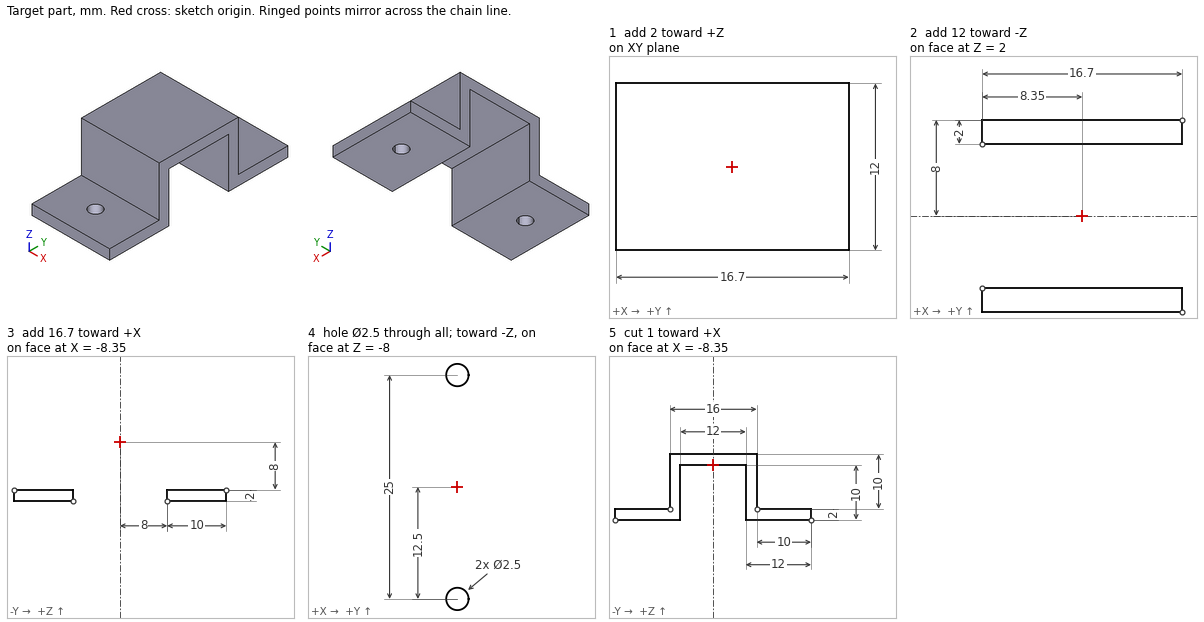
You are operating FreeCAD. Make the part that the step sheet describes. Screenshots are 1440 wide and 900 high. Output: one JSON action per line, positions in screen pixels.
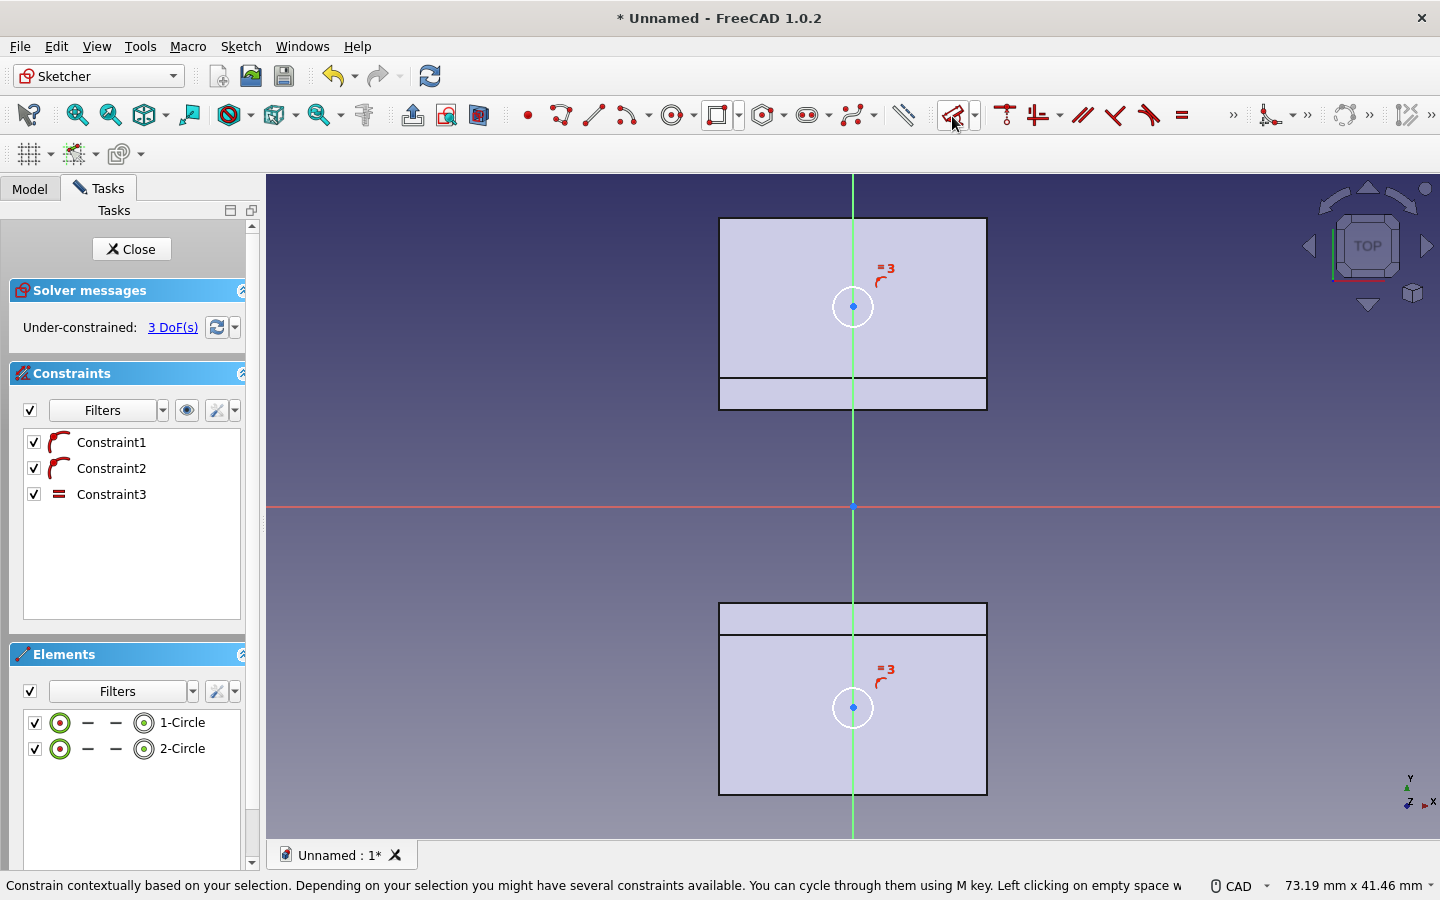
{"action": "left_click", "coordinate": [867, 694]}
{"action": "left_click", "coordinate": [890, 671]}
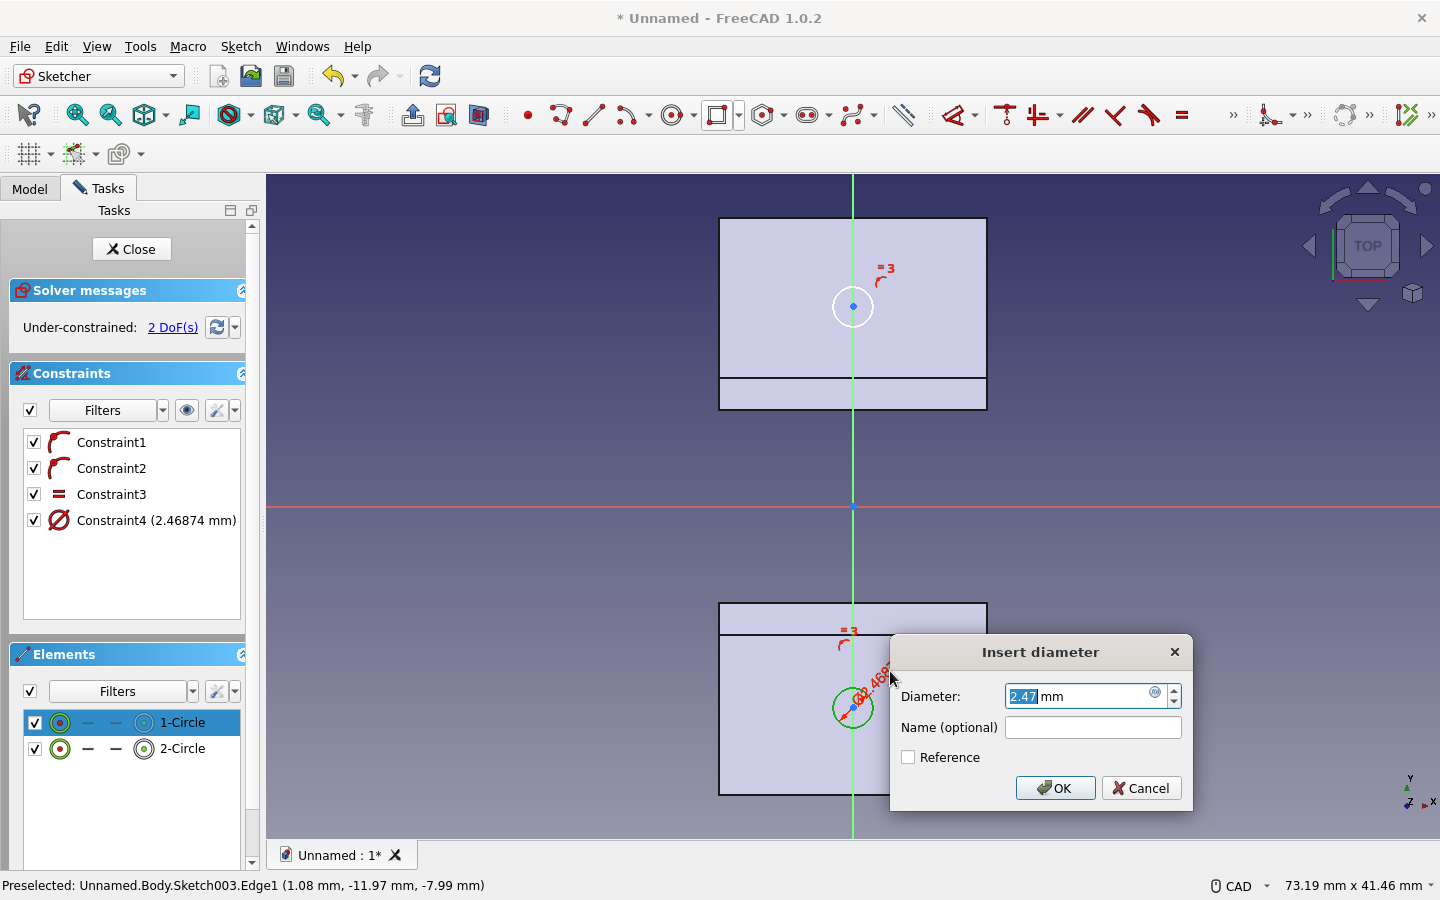
{"action": "type", "text": "2.5"}
{"action": "key", "text": "Return"}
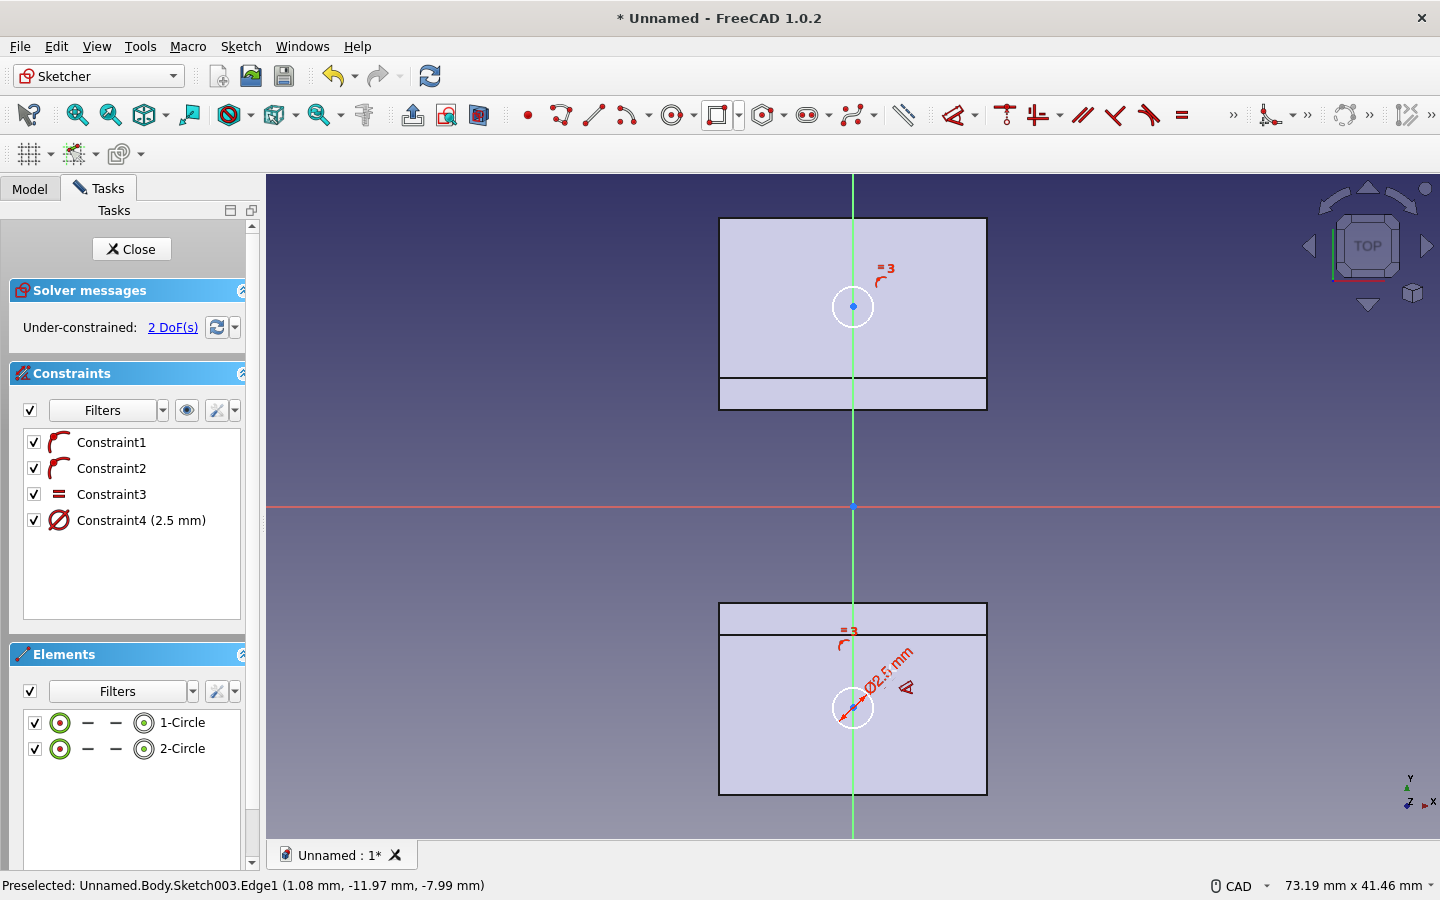
{"action": "left_click", "coordinate": [853, 708]}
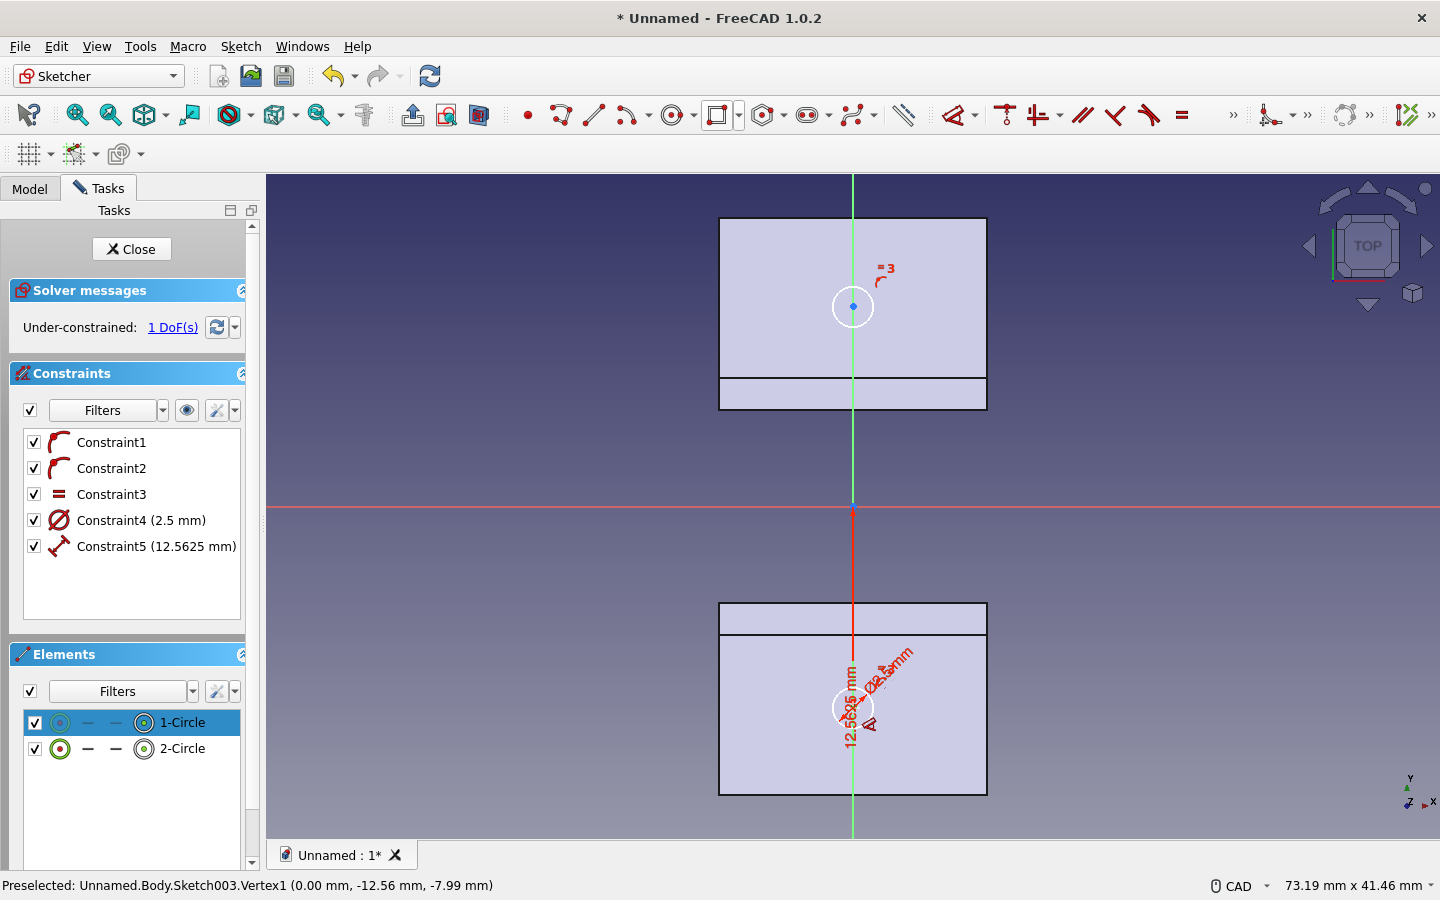
{"action": "left_click", "coordinate": [853, 307]}
{"action": "left_click", "coordinate": [887, 415]}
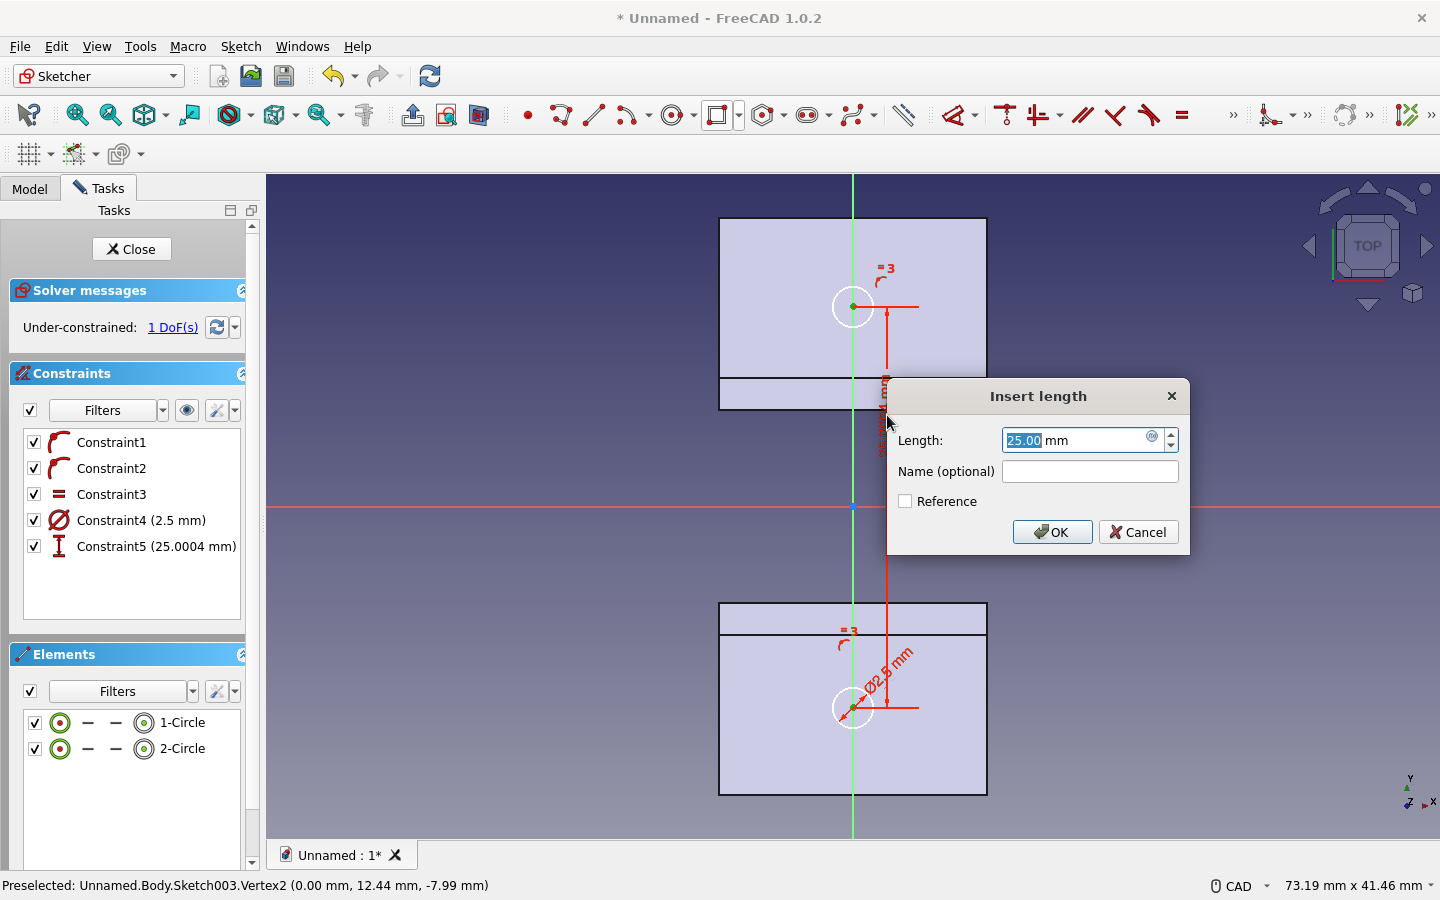
{"action": "type", "text": "25"}
{"action": "key", "text": "Return"}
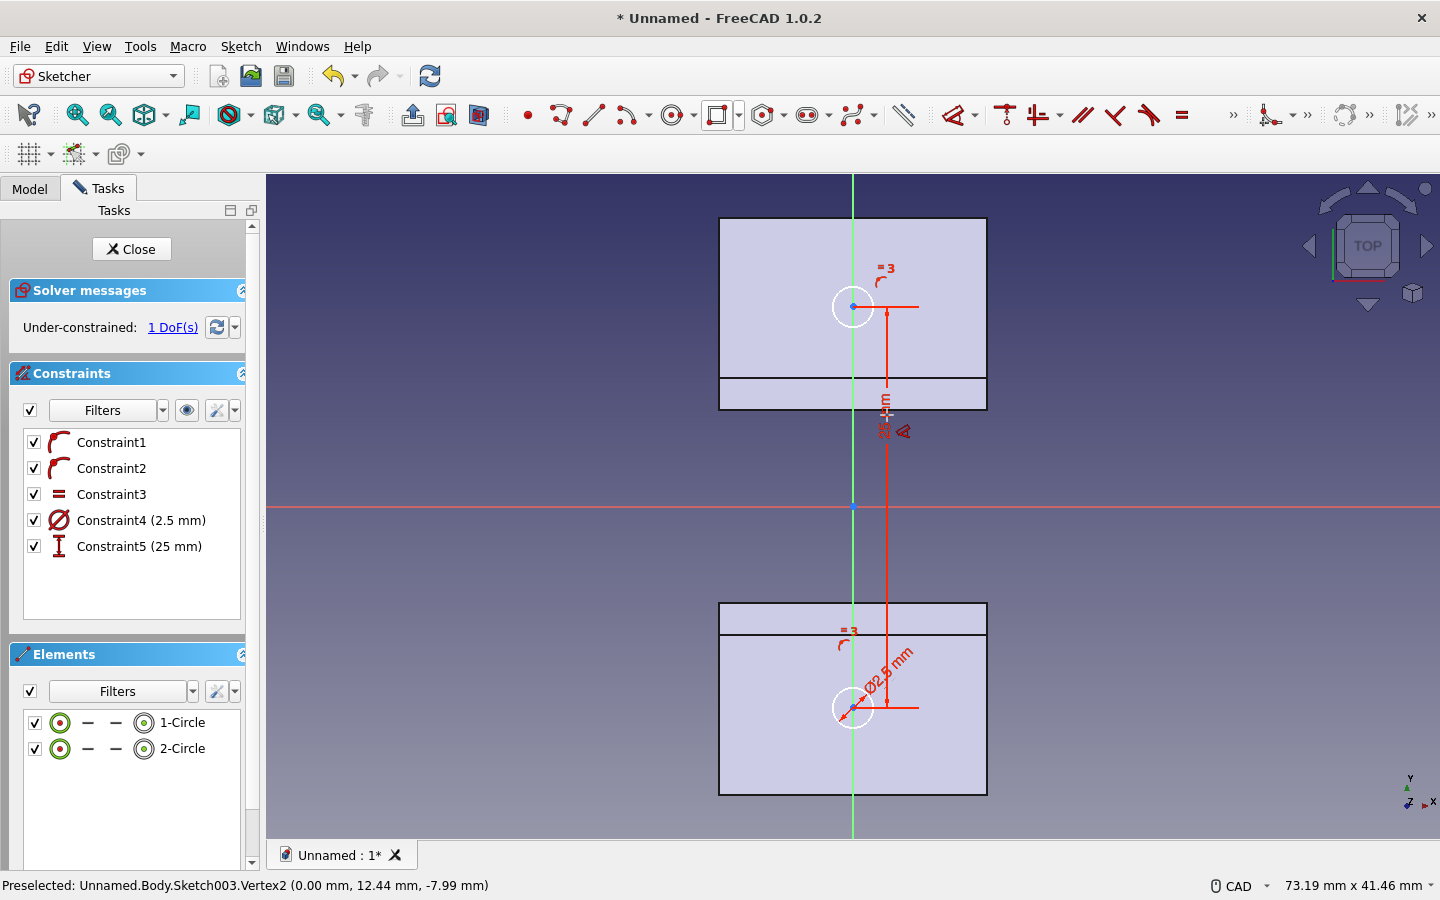
{"action": "left_click", "coordinate": [853, 708]}
{"action": "left_click", "coordinate": [887, 607]}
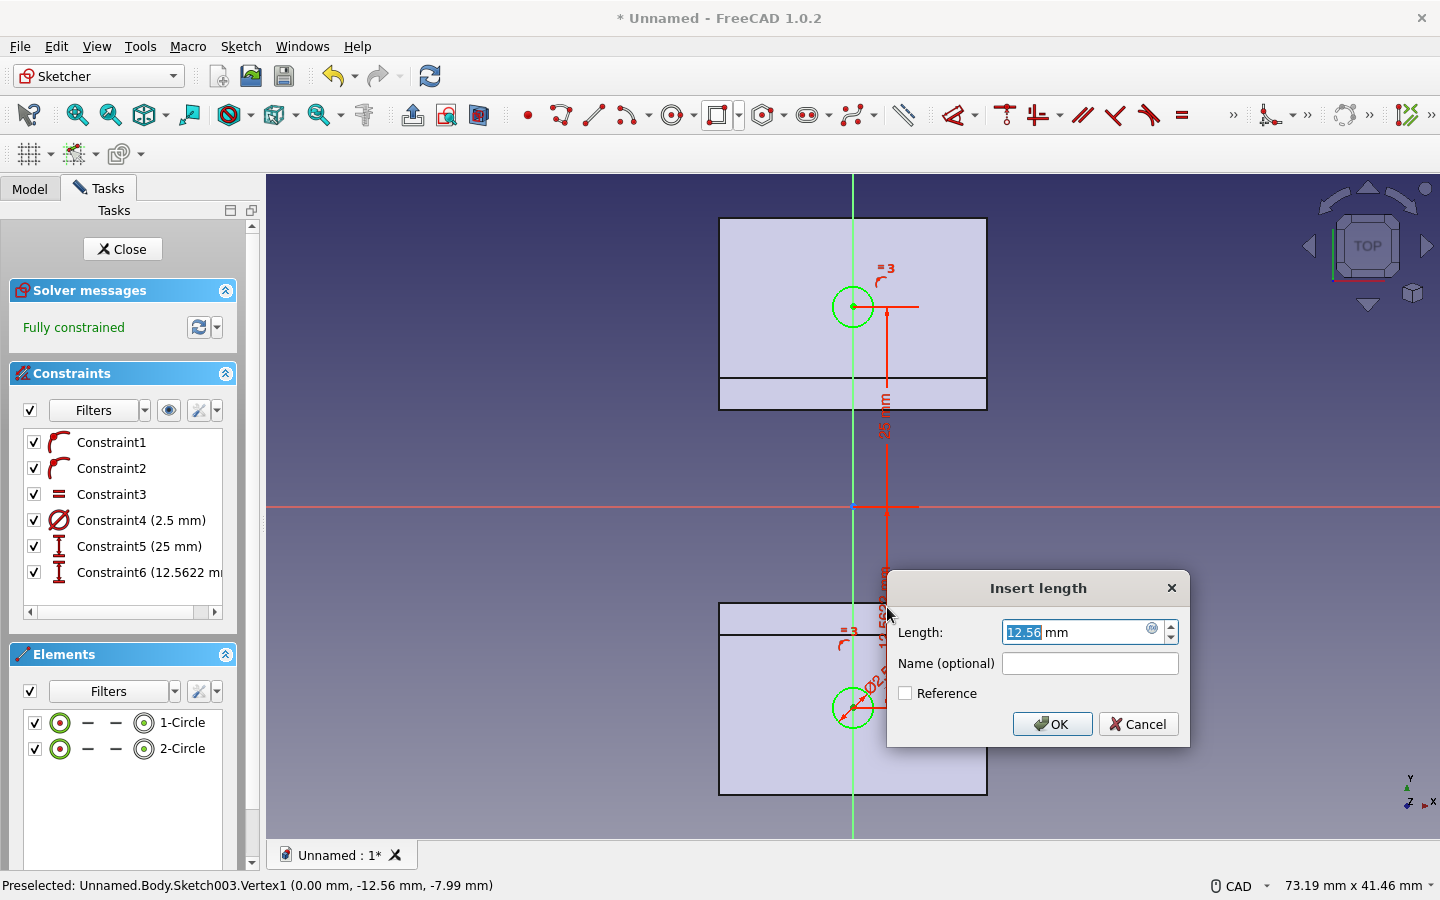
{"action": "type", "text": "12.5"}
{"action": "key", "text": "Return"}
{"action": "key", "text": "Escape"}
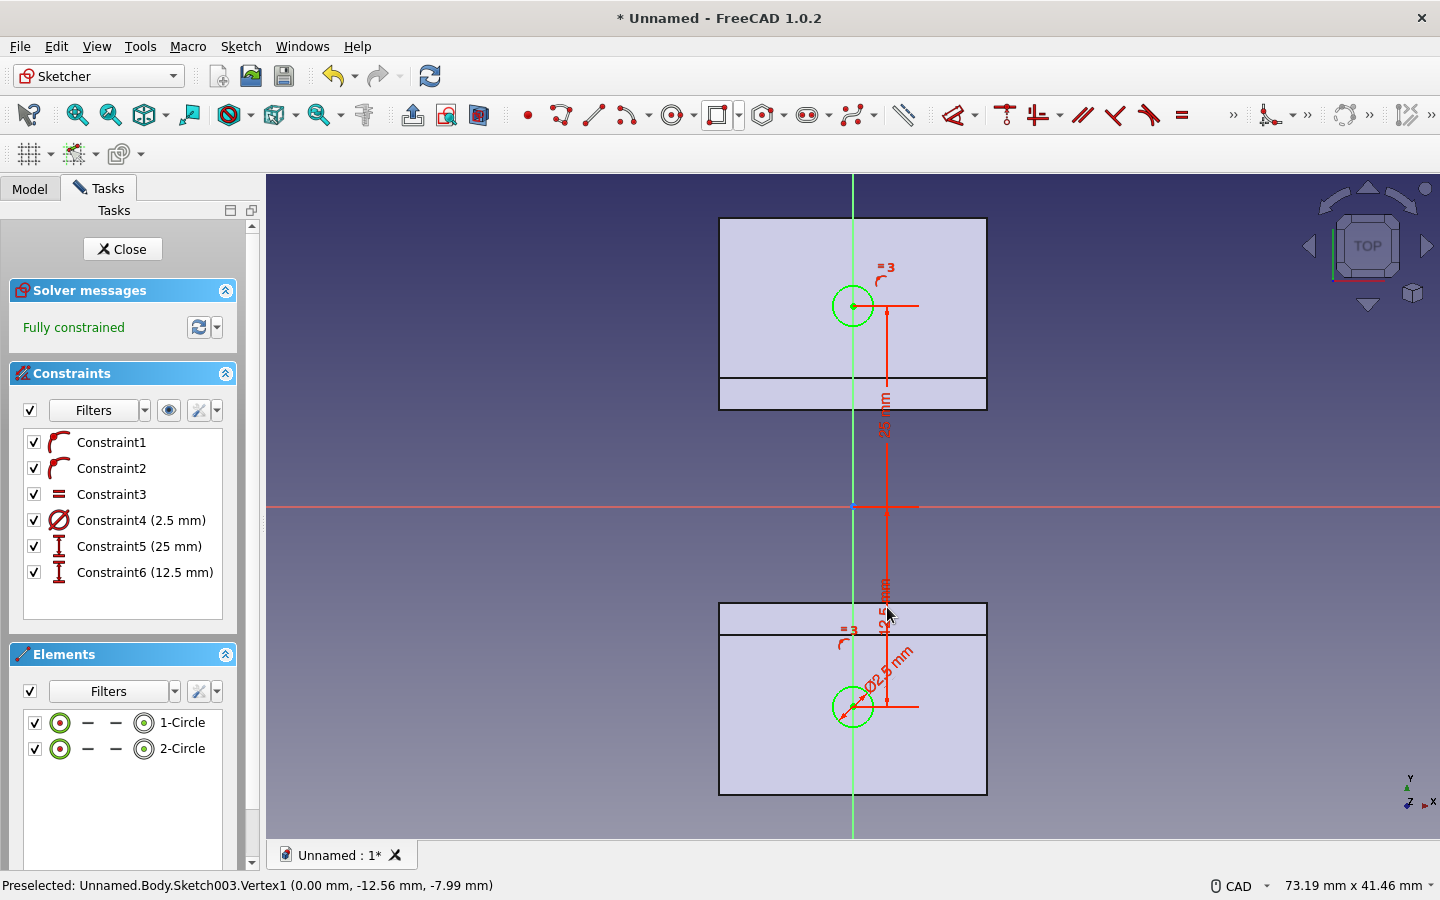
{"action": "left_click", "coordinate": [123, 249]}